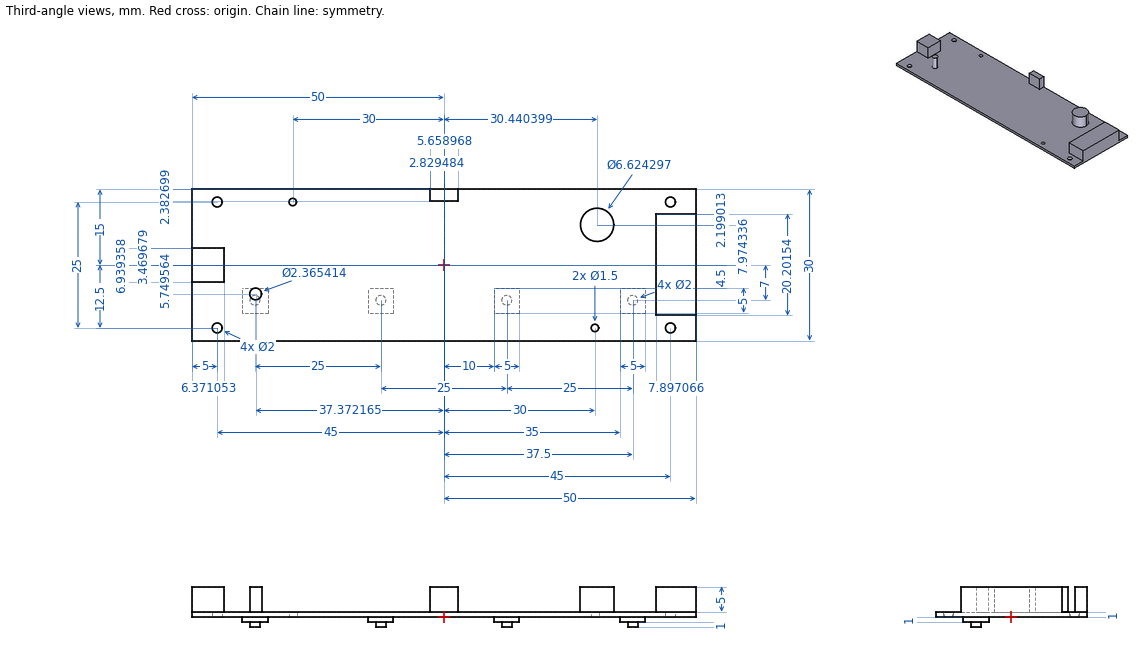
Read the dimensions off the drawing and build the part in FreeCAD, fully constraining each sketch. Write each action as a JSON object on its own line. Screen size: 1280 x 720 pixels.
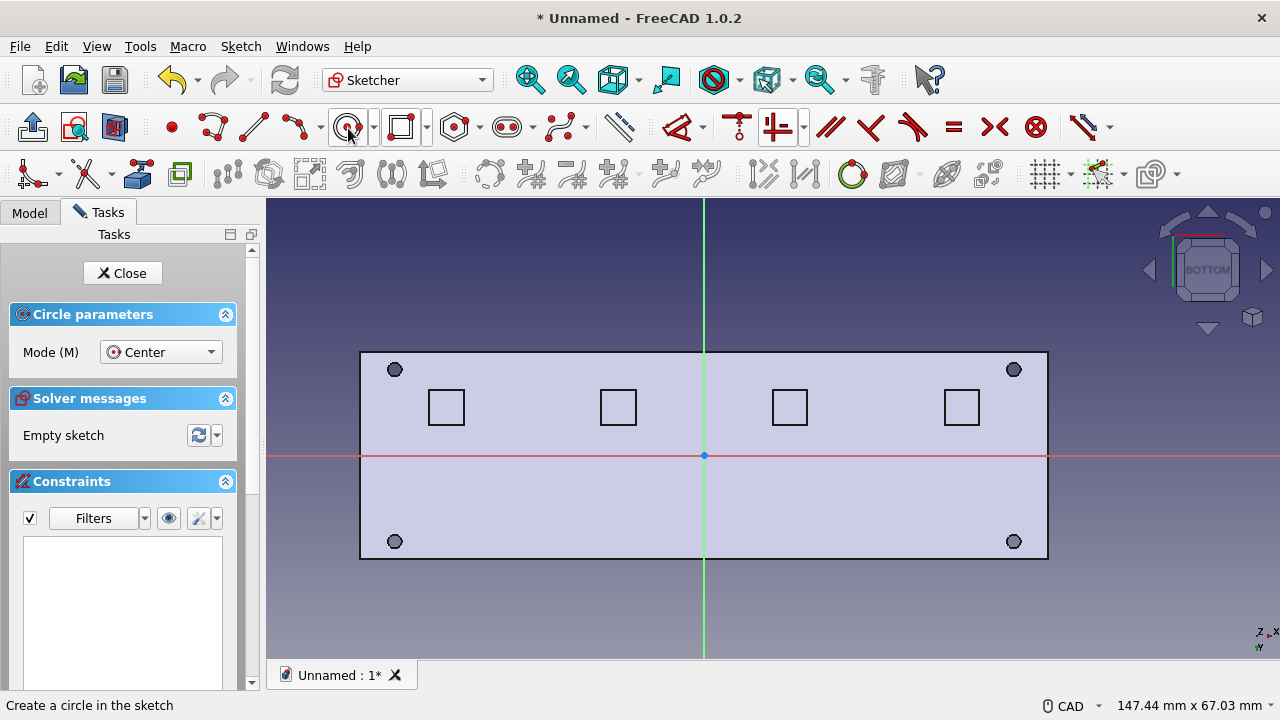
{"action": "scroll", "coordinate": [962, 407], "scroll_direction": "up", "scroll_amount": 6}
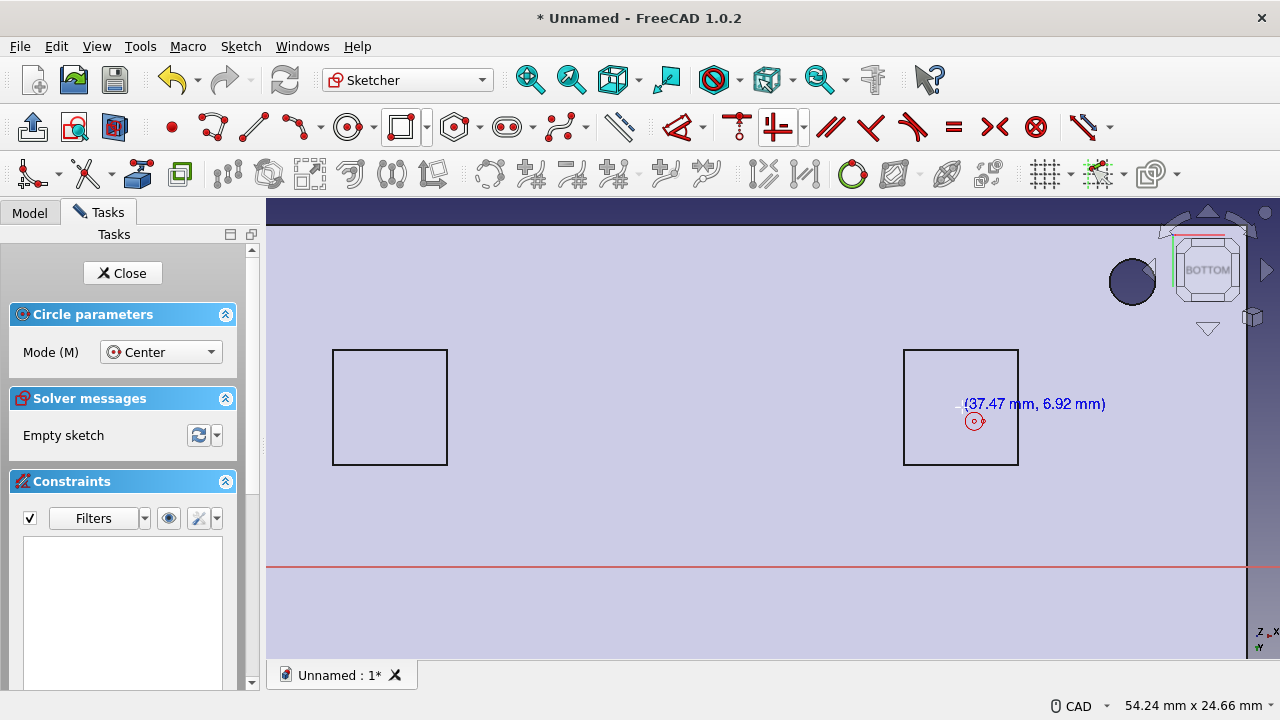
{"action": "left_click", "coordinate": [961, 407]}
{"action": "left_click", "coordinate": [977, 391]}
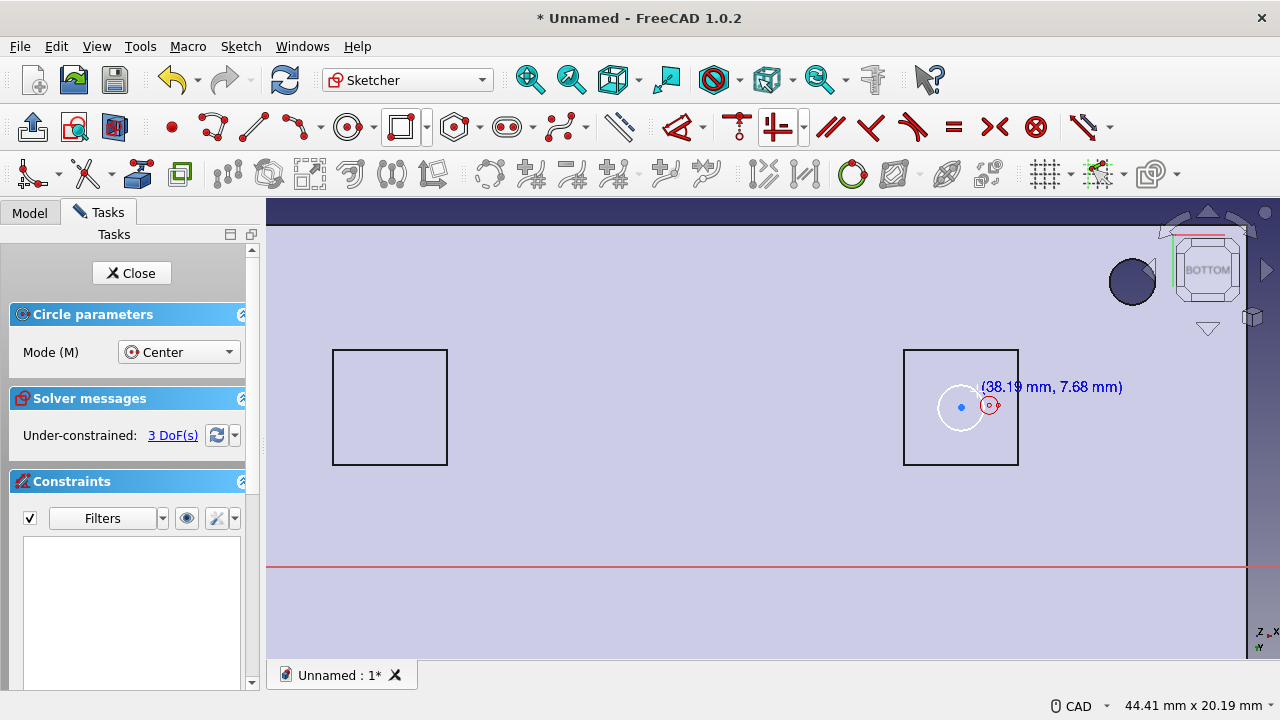
{"action": "left_click", "coordinate": [390, 407]}
{"action": "left_click", "coordinate": [406, 391]}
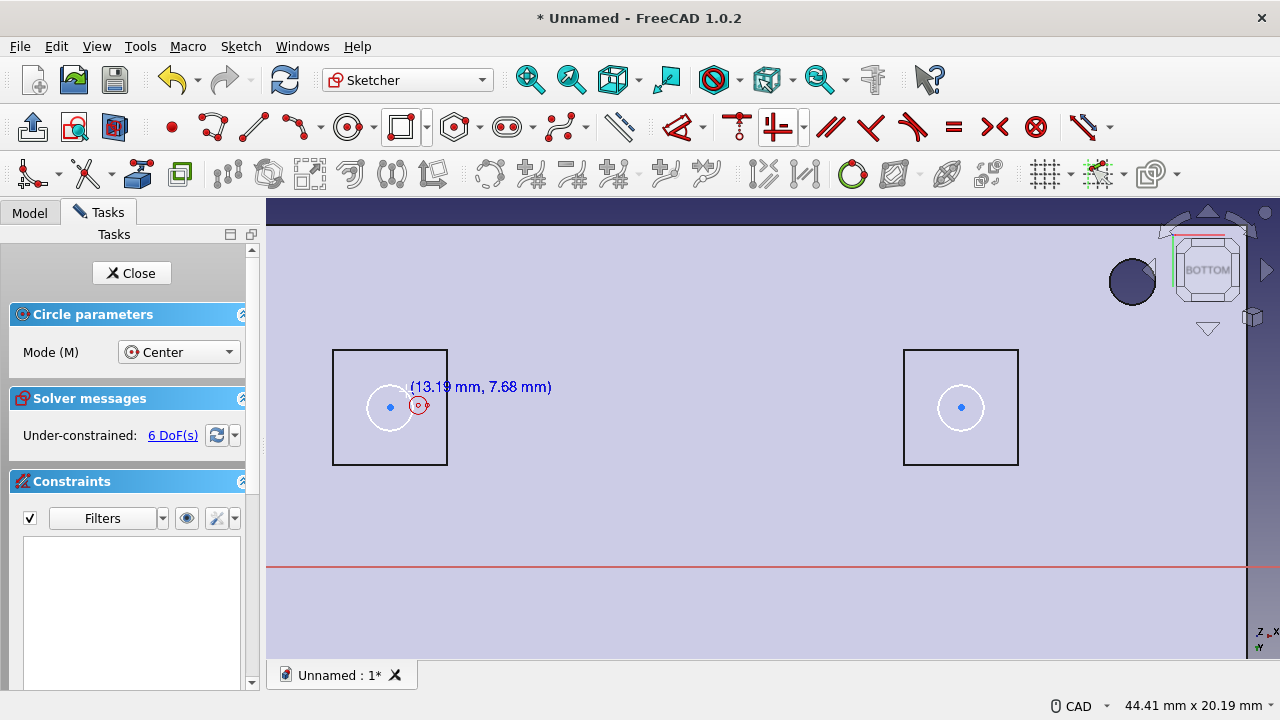
{"action": "scroll", "coordinate": [963, 408], "scroll_direction": "down", "scroll_amount": 6}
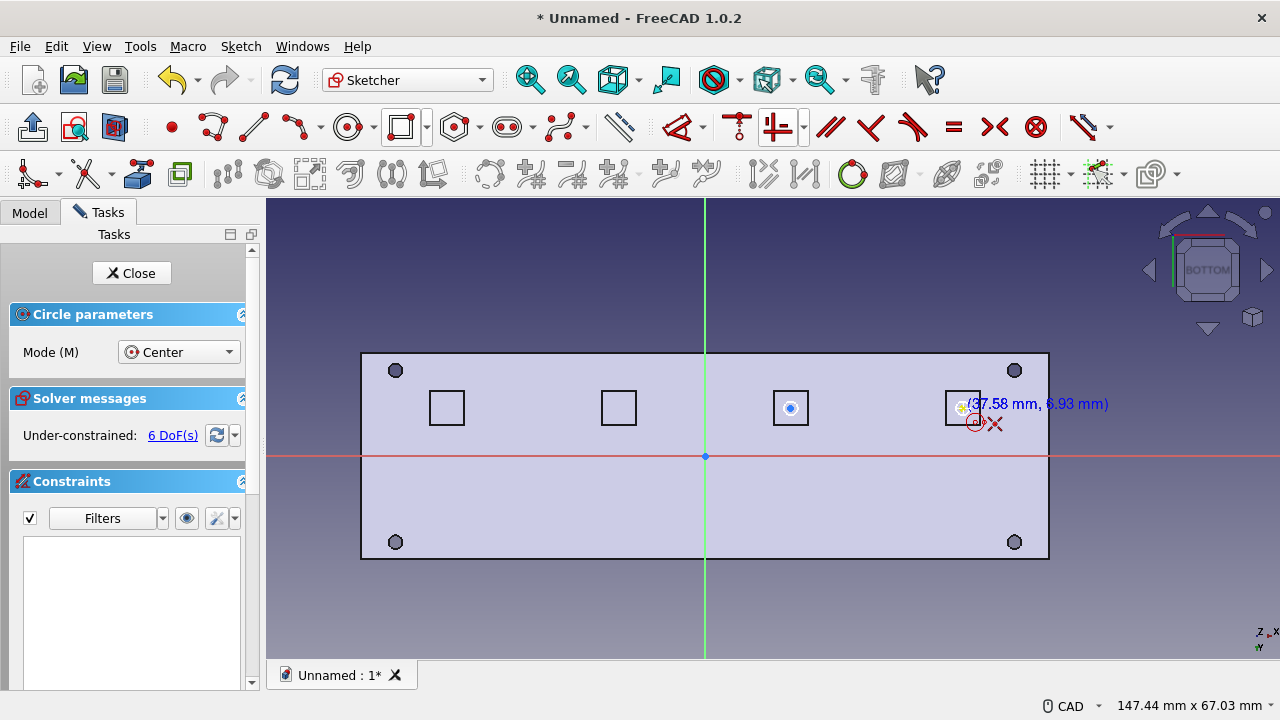
{"action": "scroll", "coordinate": [619, 408], "scroll_direction": "up", "scroll_amount": 6}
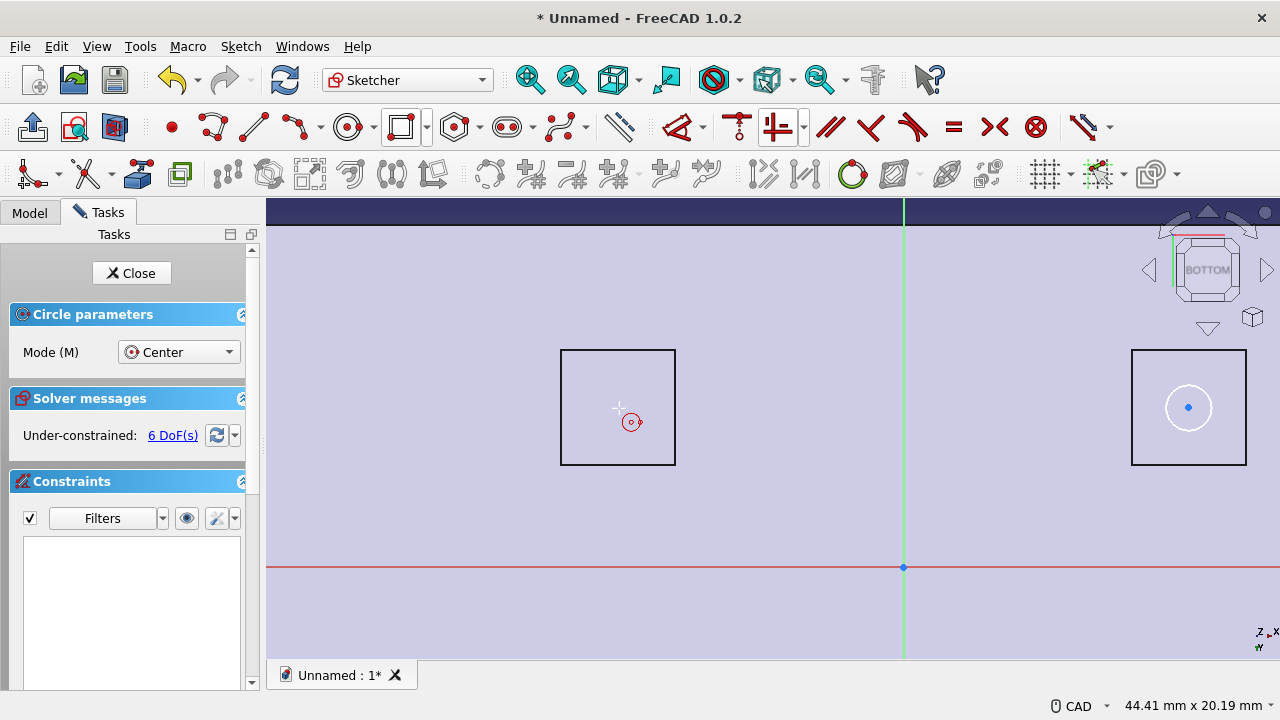
{"action": "left_click", "coordinate": [618, 407]}
{"action": "left_click", "coordinate": [635, 391]}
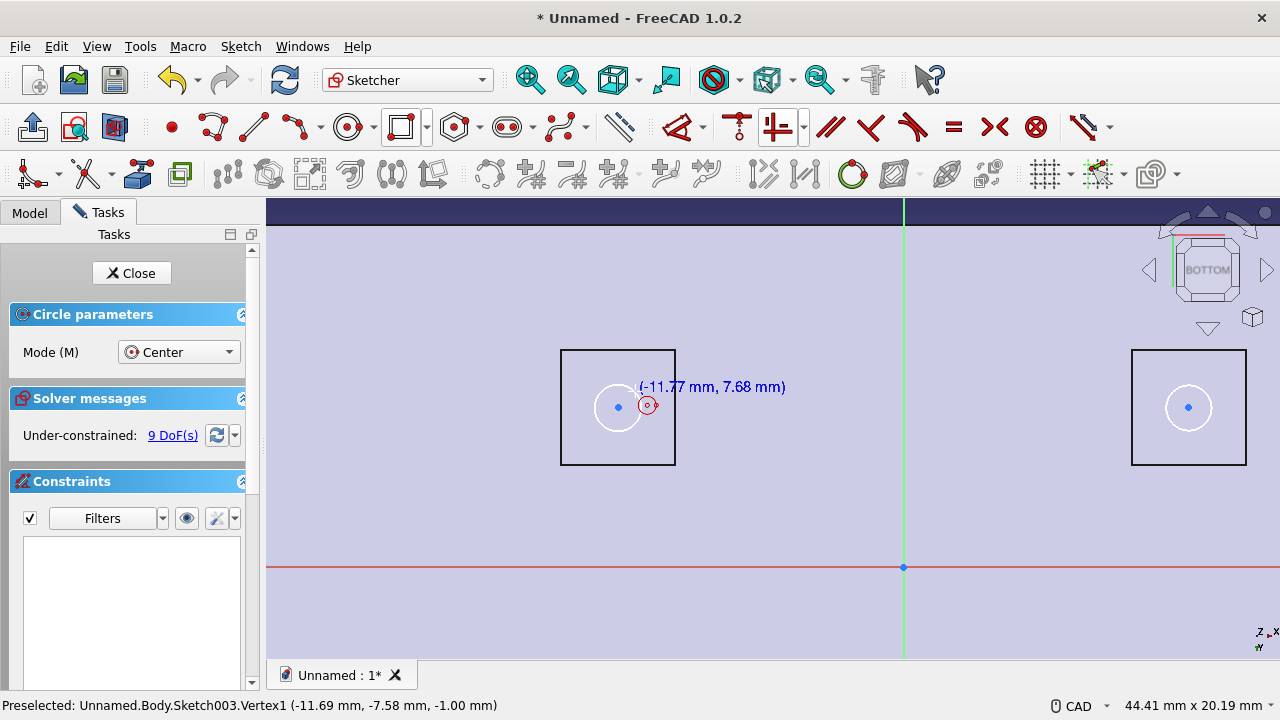
{"action": "scroll", "coordinate": [619, 408], "scroll_direction": "down", "scroll_amount": 6}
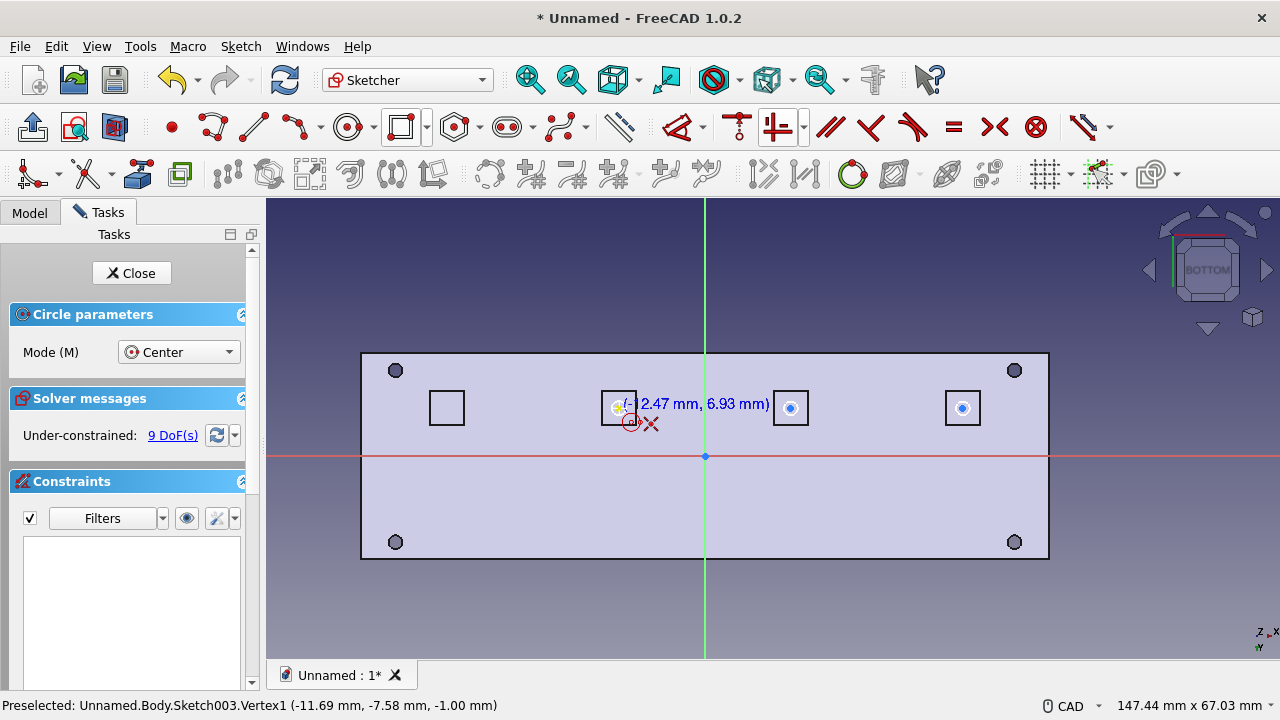
{"action": "scroll", "coordinate": [447, 408], "scroll_direction": "up", "scroll_amount": 6}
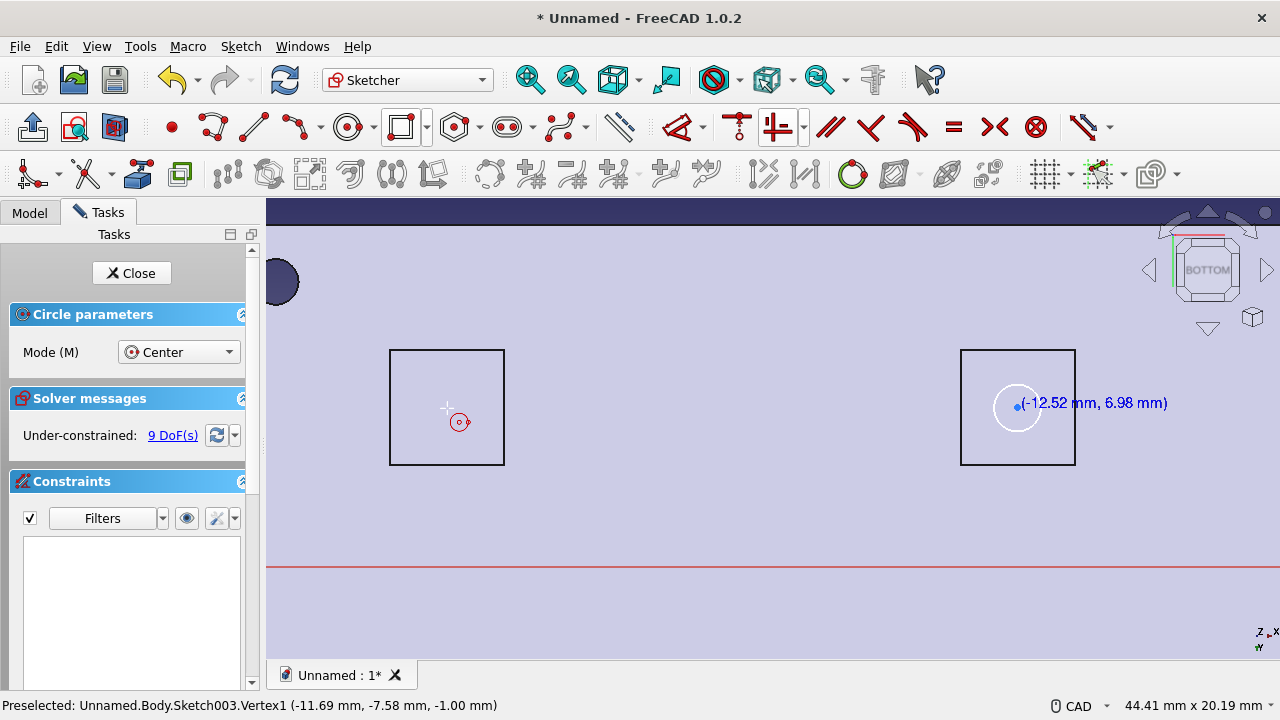
{"action": "left_click", "coordinate": [447, 407]}
{"action": "left_click", "coordinate": [463, 391]}
{"action": "key", "text": "Escape"}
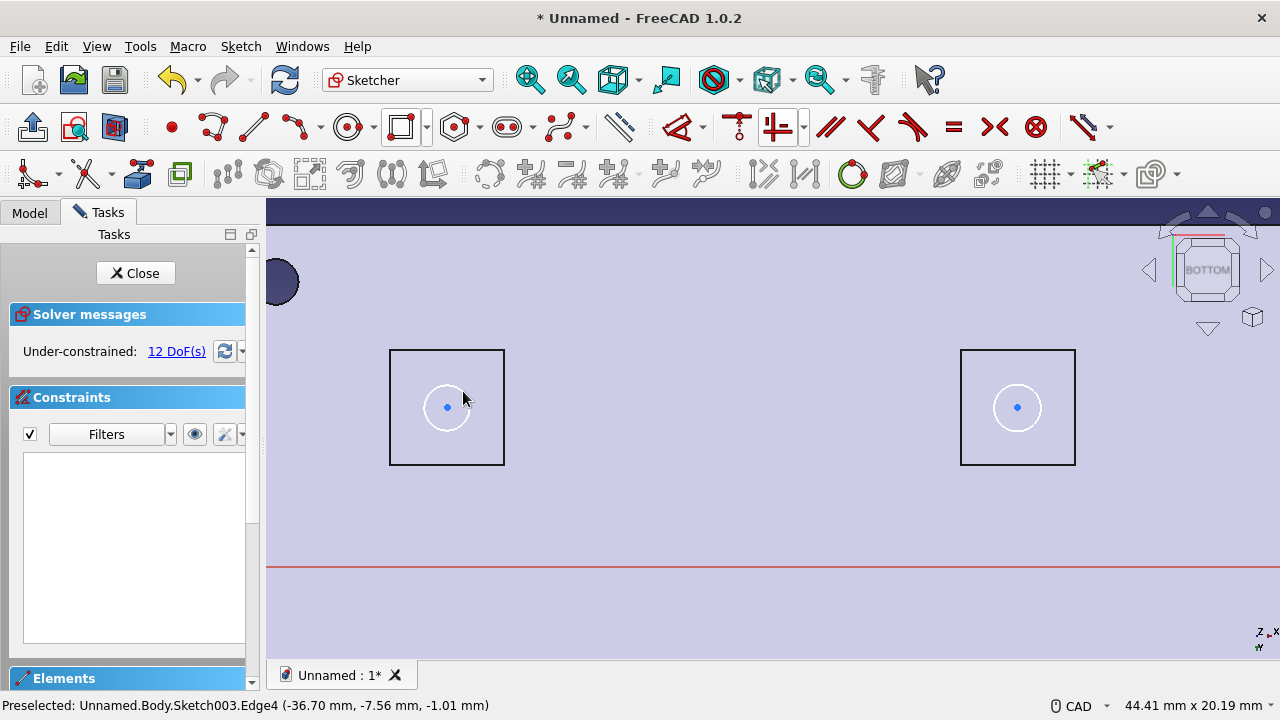
{"action": "scroll", "coordinate": [446, 408], "scroll_direction": "down", "scroll_amount": 6}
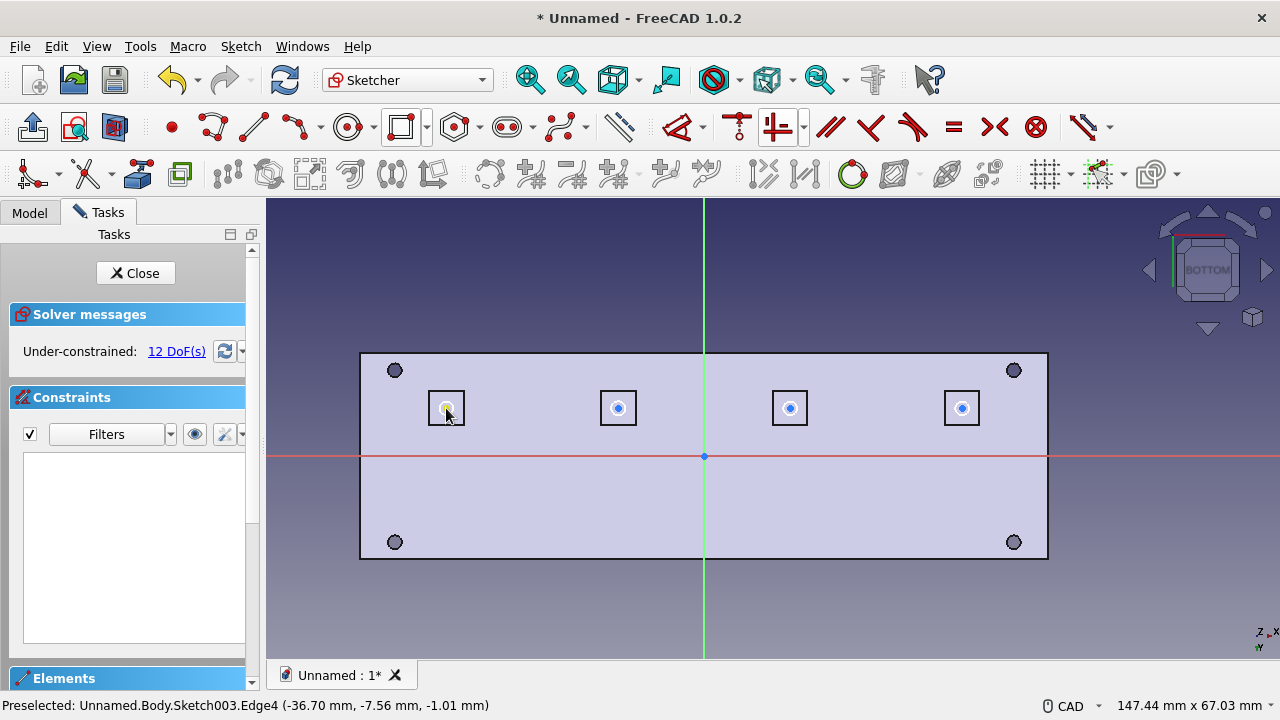
{"action": "scroll", "coordinate": [967, 403], "scroll_direction": "up", "scroll_amount": 4}